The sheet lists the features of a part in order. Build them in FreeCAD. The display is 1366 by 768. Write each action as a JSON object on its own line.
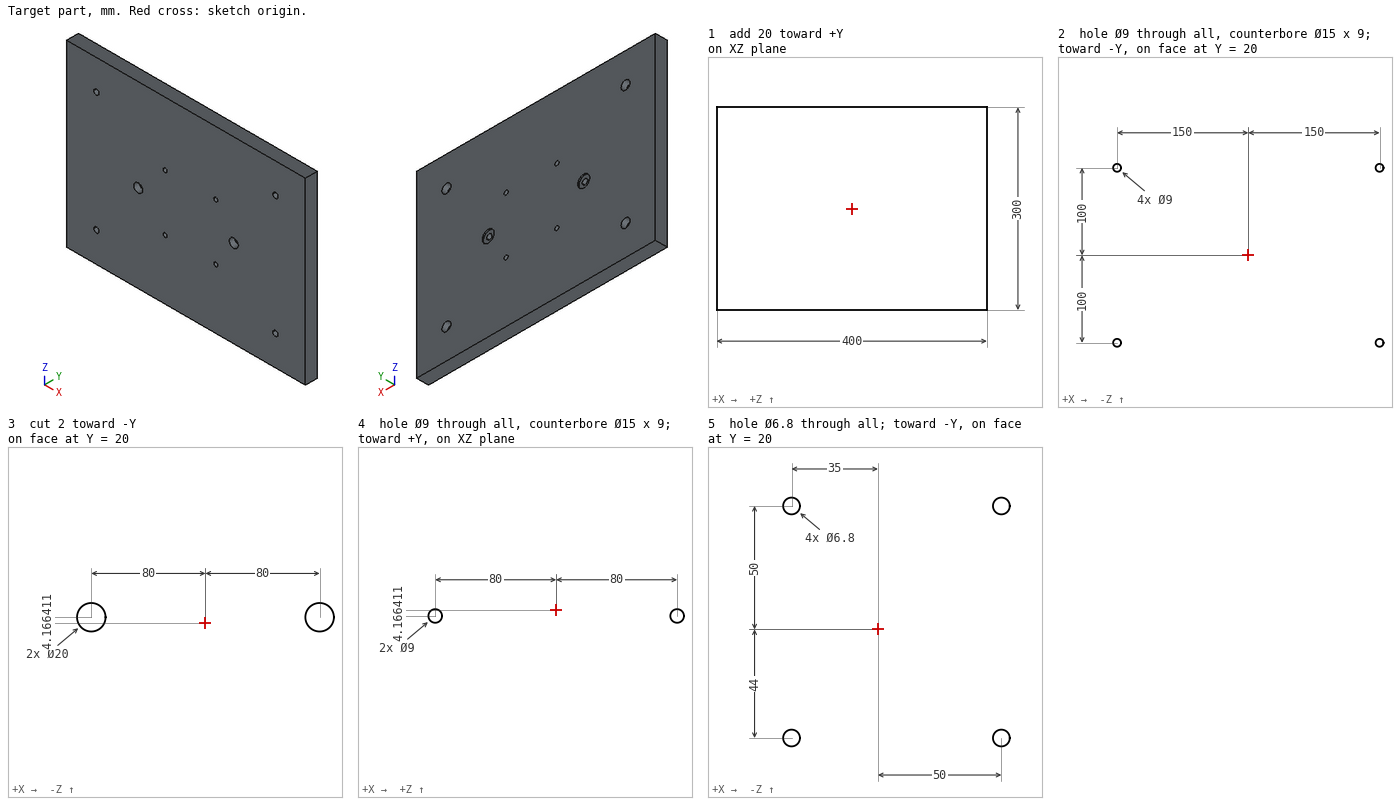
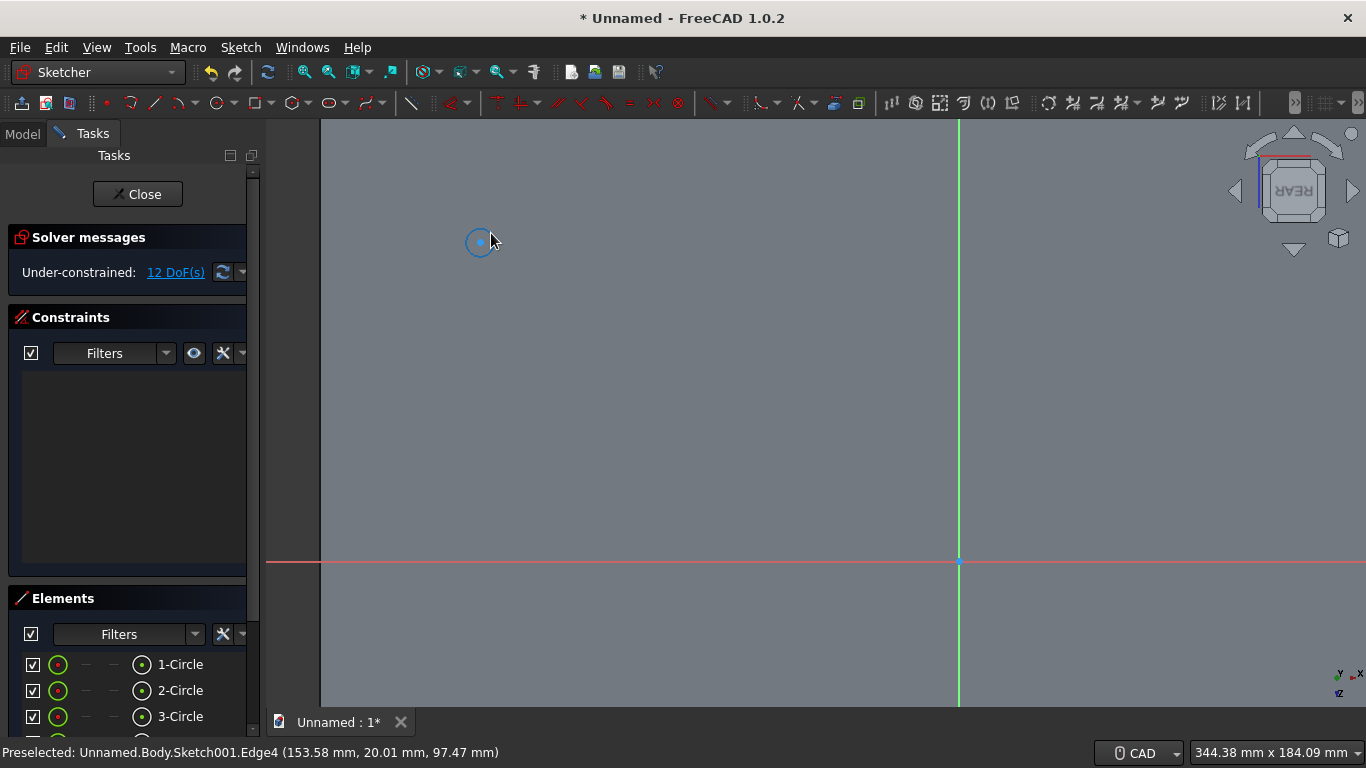
{"action": "left_click", "coordinate": [490, 233]}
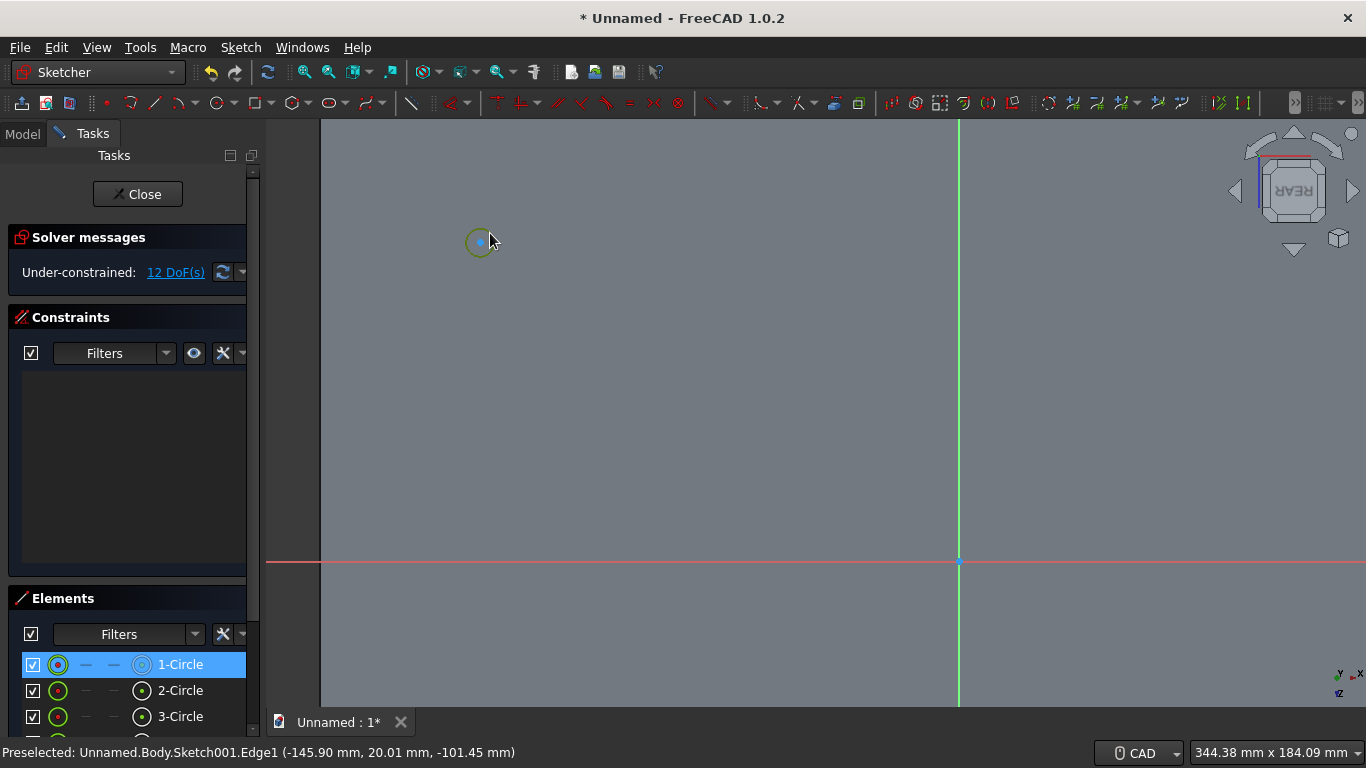
{"action": "scroll", "coordinate": [490, 232], "scroll_direction": "down", "scroll_amount": 3}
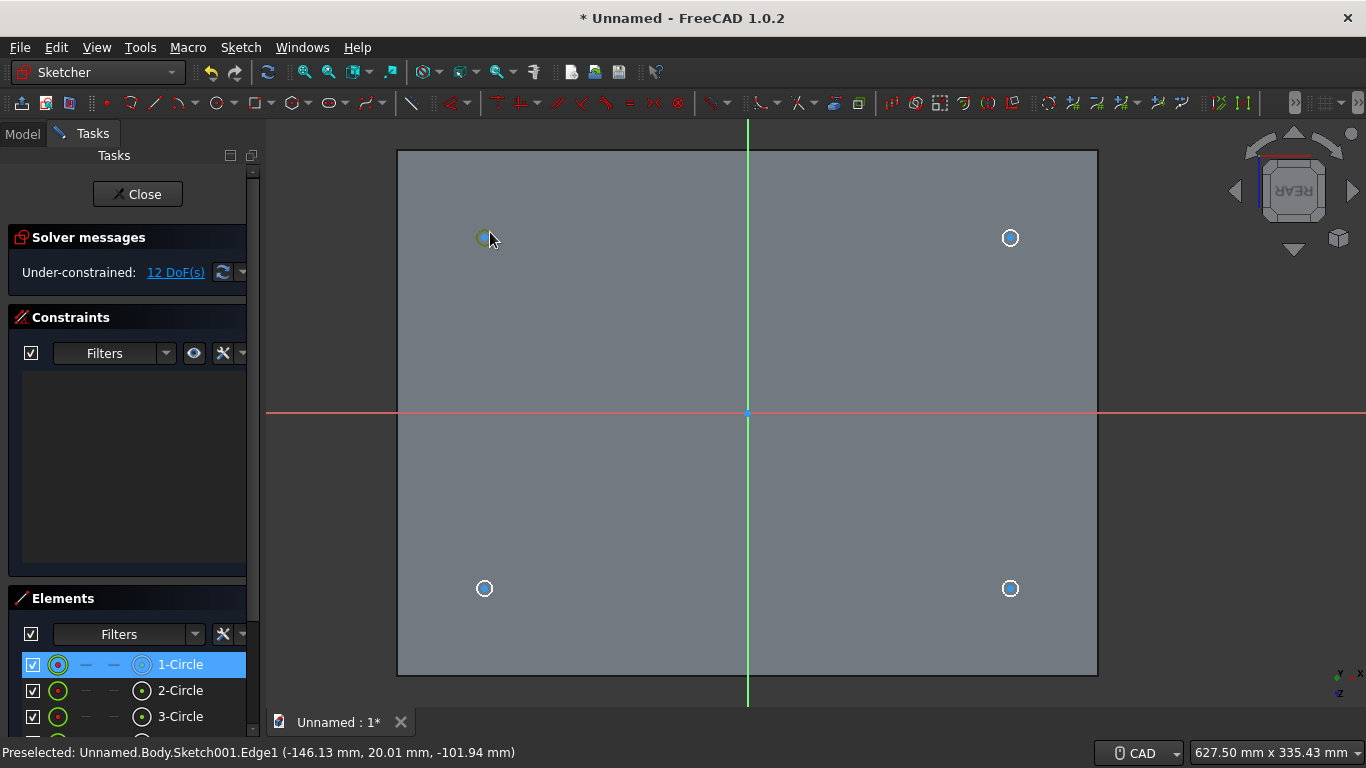
{"action": "scroll", "coordinate": [490, 583], "scroll_direction": "up", "scroll_amount": 3}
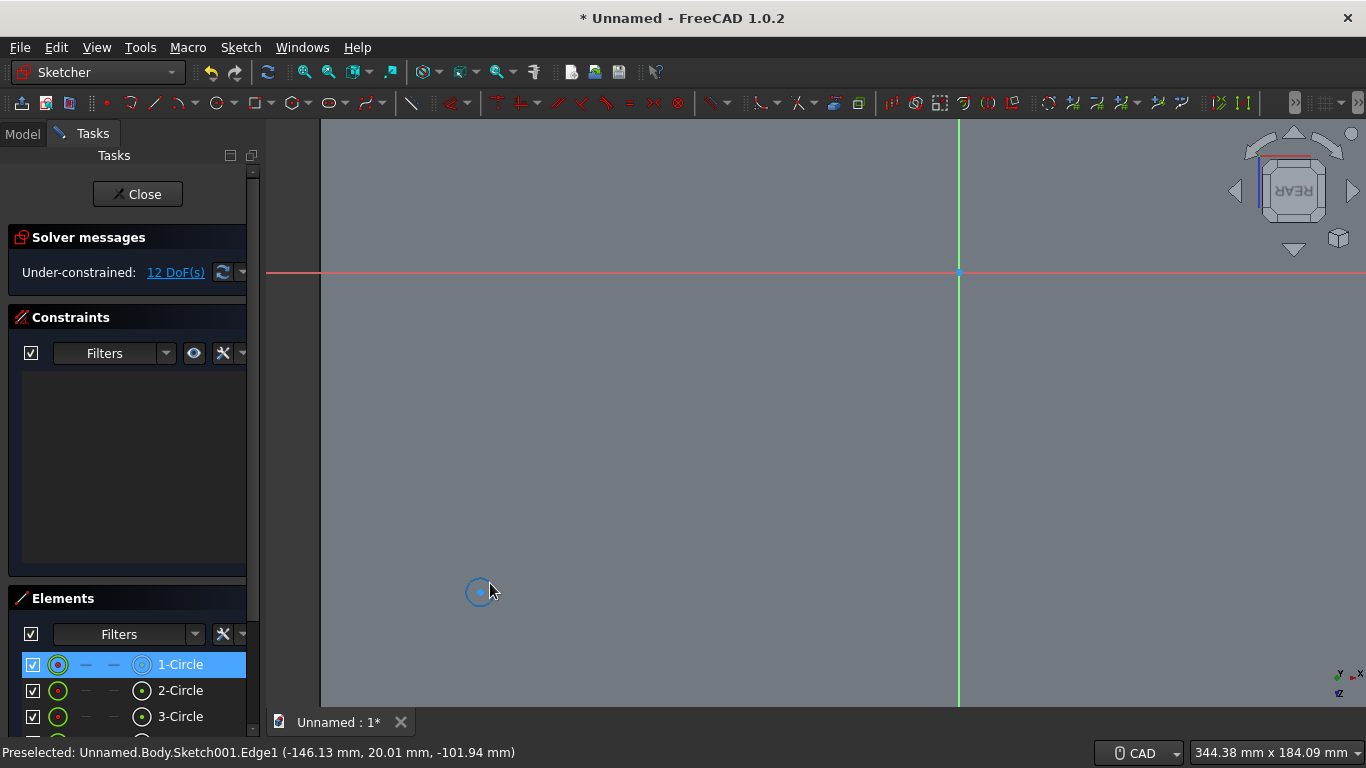
{"action": "left_click", "coordinate": [490, 582]}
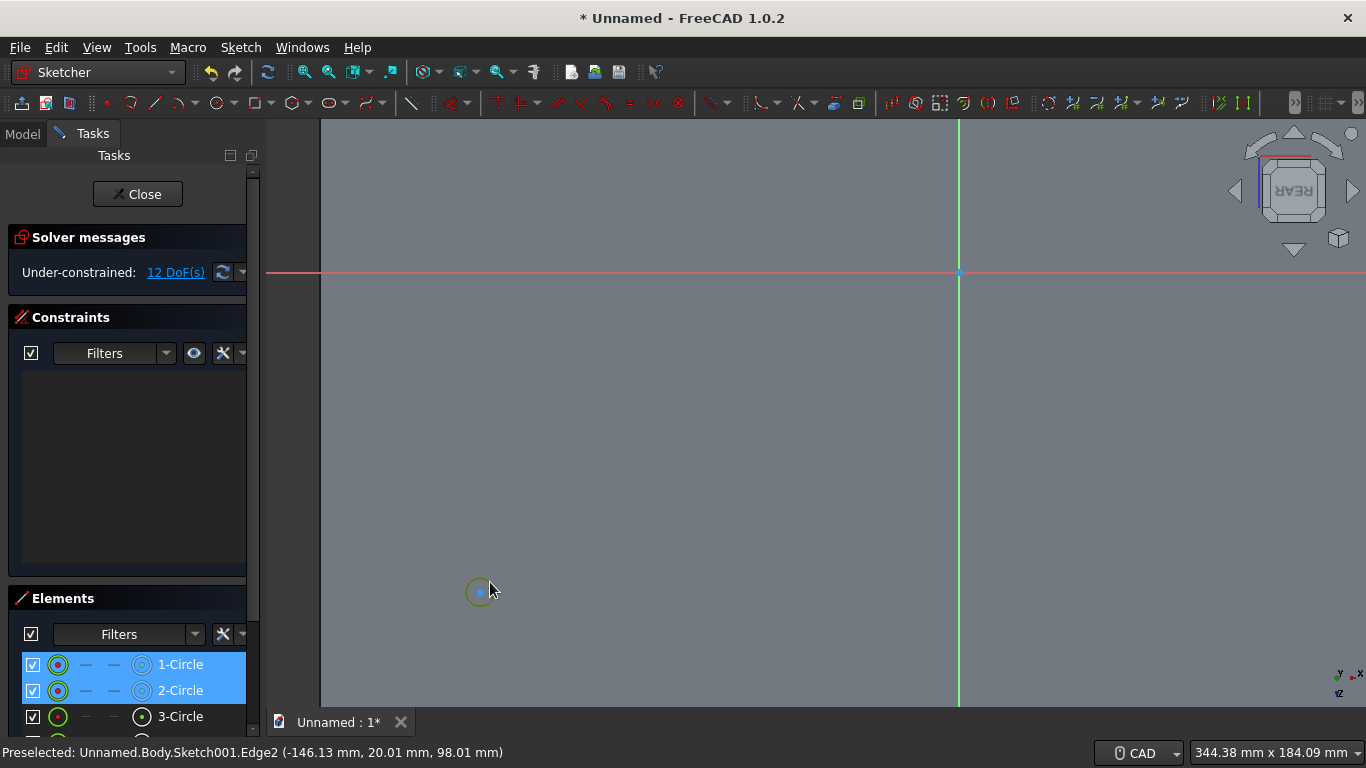
{"action": "scroll", "coordinate": [490, 584], "scroll_direction": "down", "scroll_amount": 3}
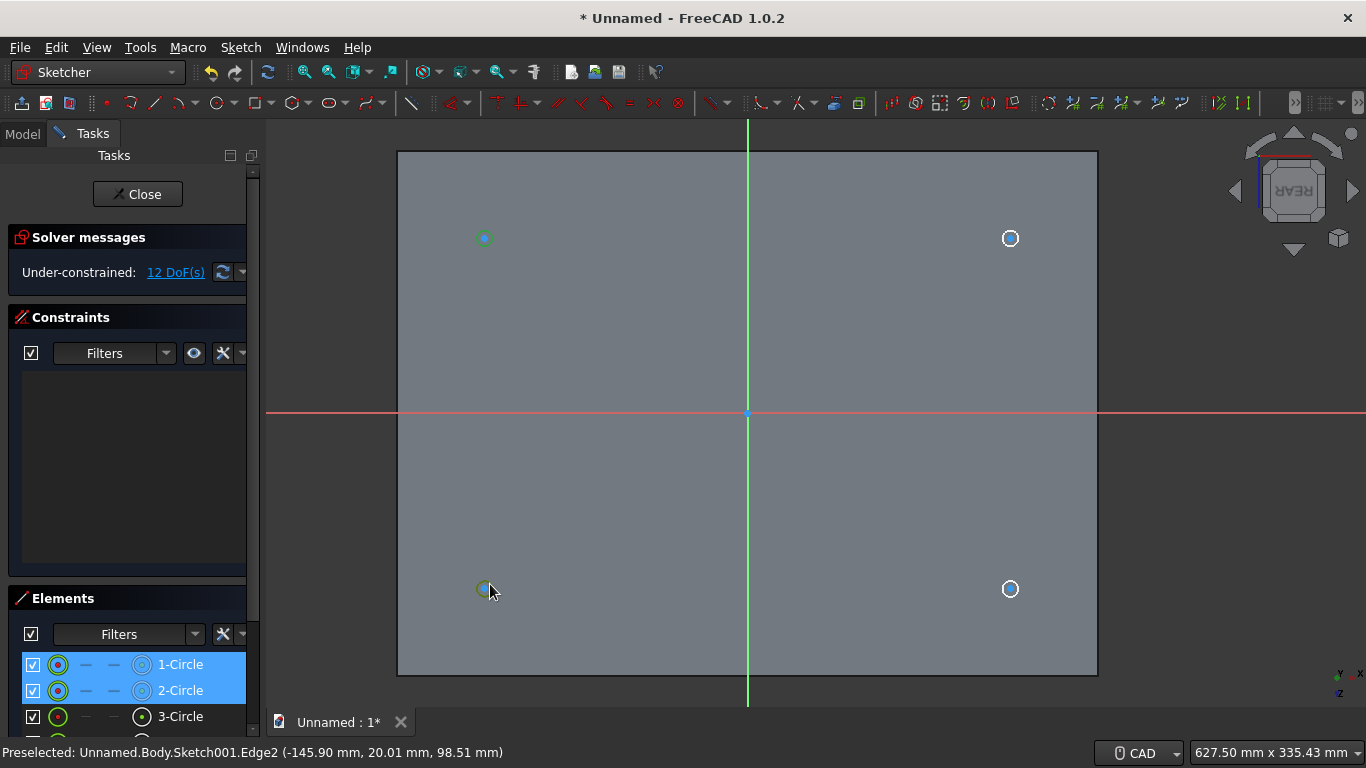
{"action": "scroll", "coordinate": [1016, 233], "scroll_direction": "up", "scroll_amount": 3}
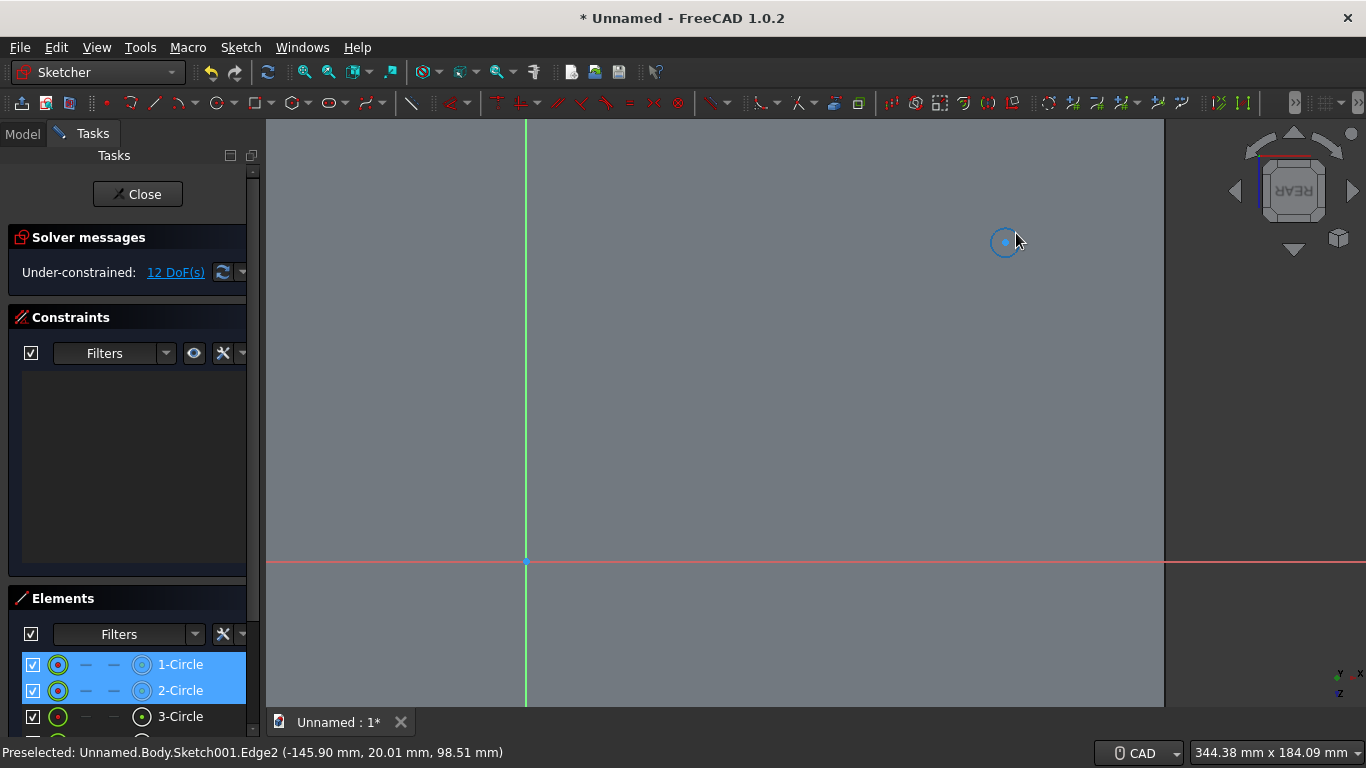
{"action": "left_click", "coordinate": [1015, 233]}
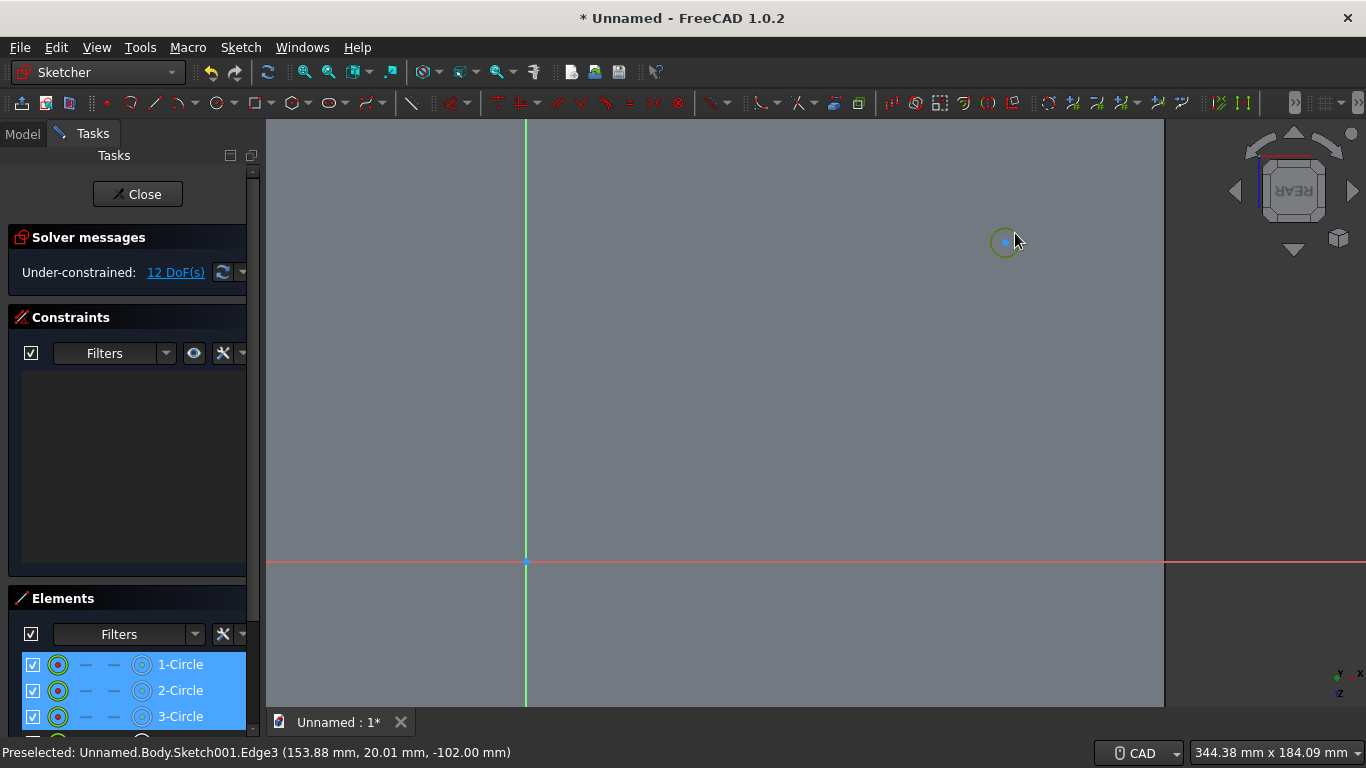
{"action": "scroll", "coordinate": [1017, 232], "scroll_direction": "down", "scroll_amount": 3}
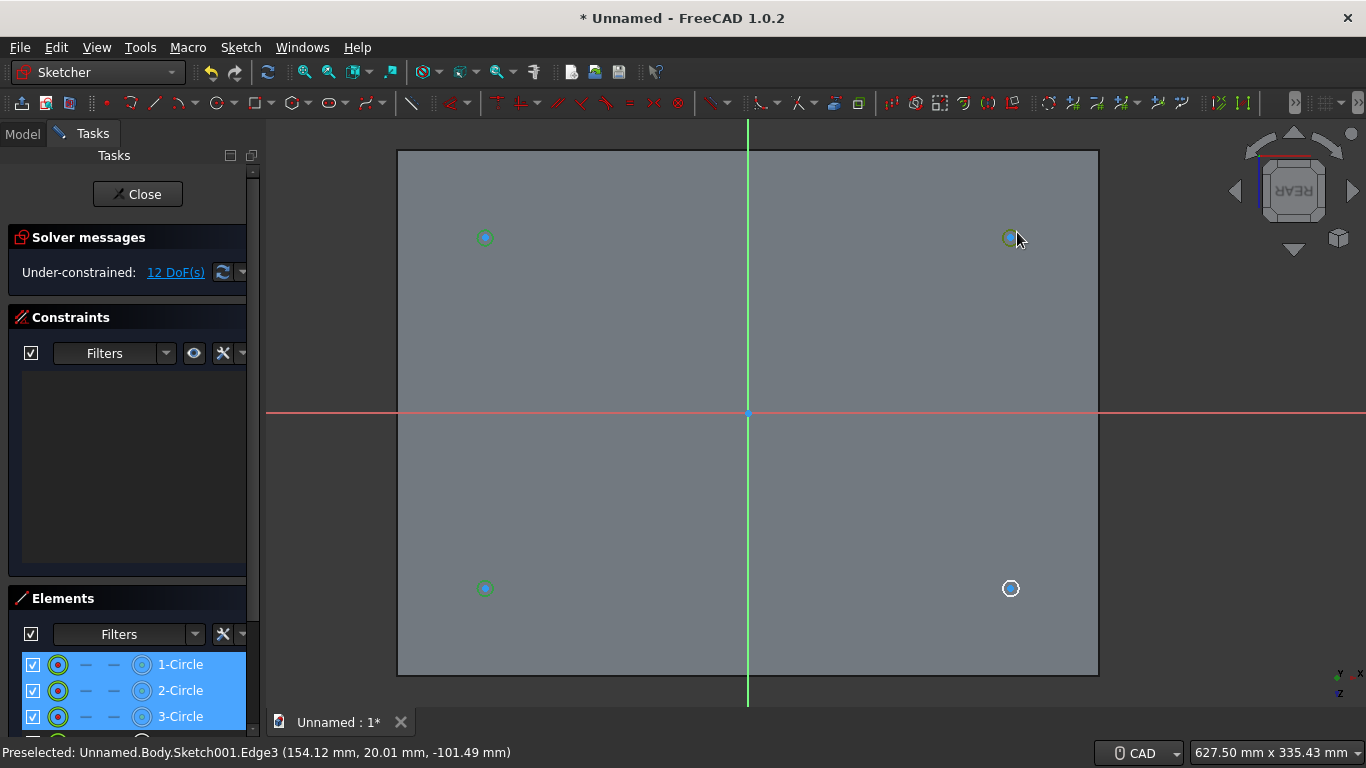
{"action": "scroll", "coordinate": [1016, 583], "scroll_direction": "up", "scroll_amount": 3}